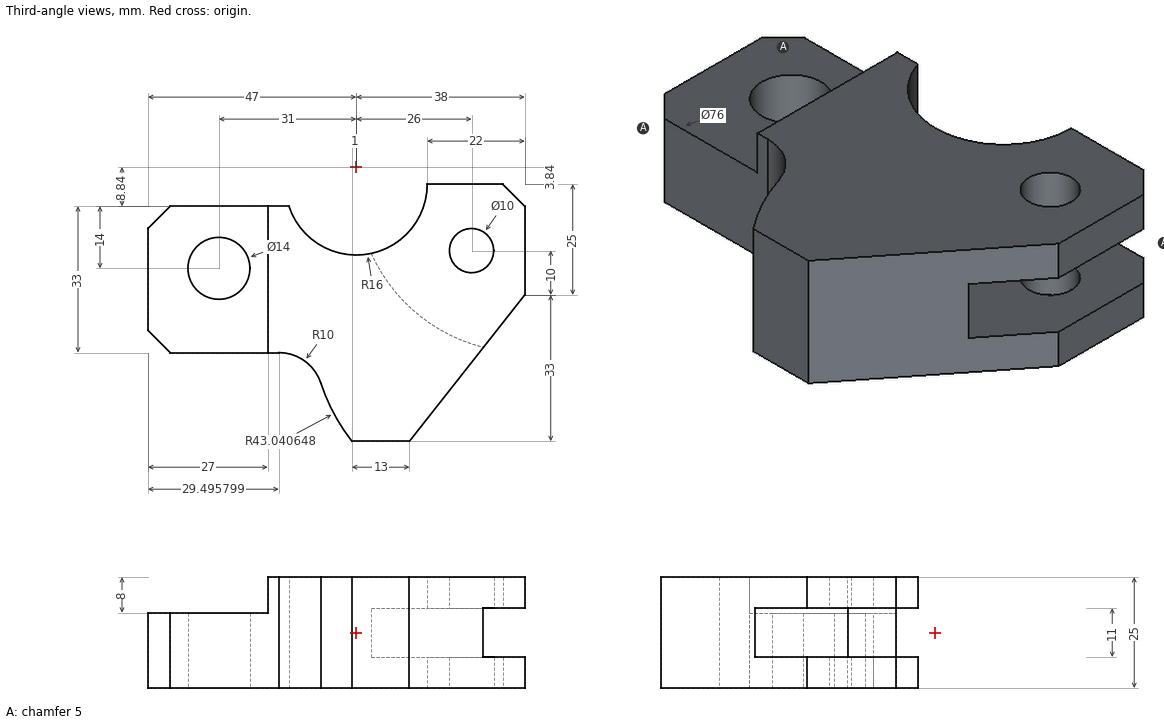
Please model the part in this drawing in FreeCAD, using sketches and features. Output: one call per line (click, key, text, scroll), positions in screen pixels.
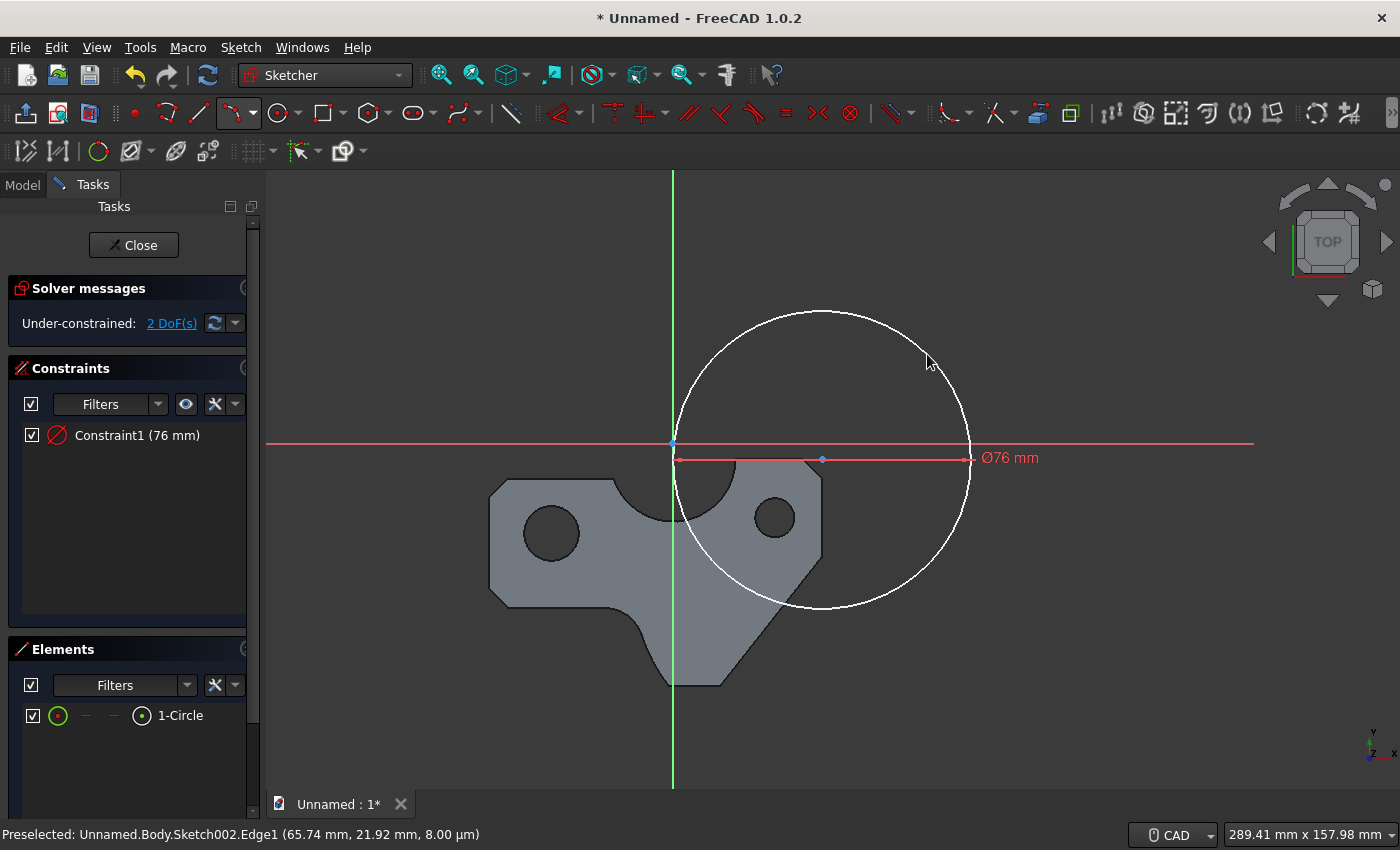
key(d)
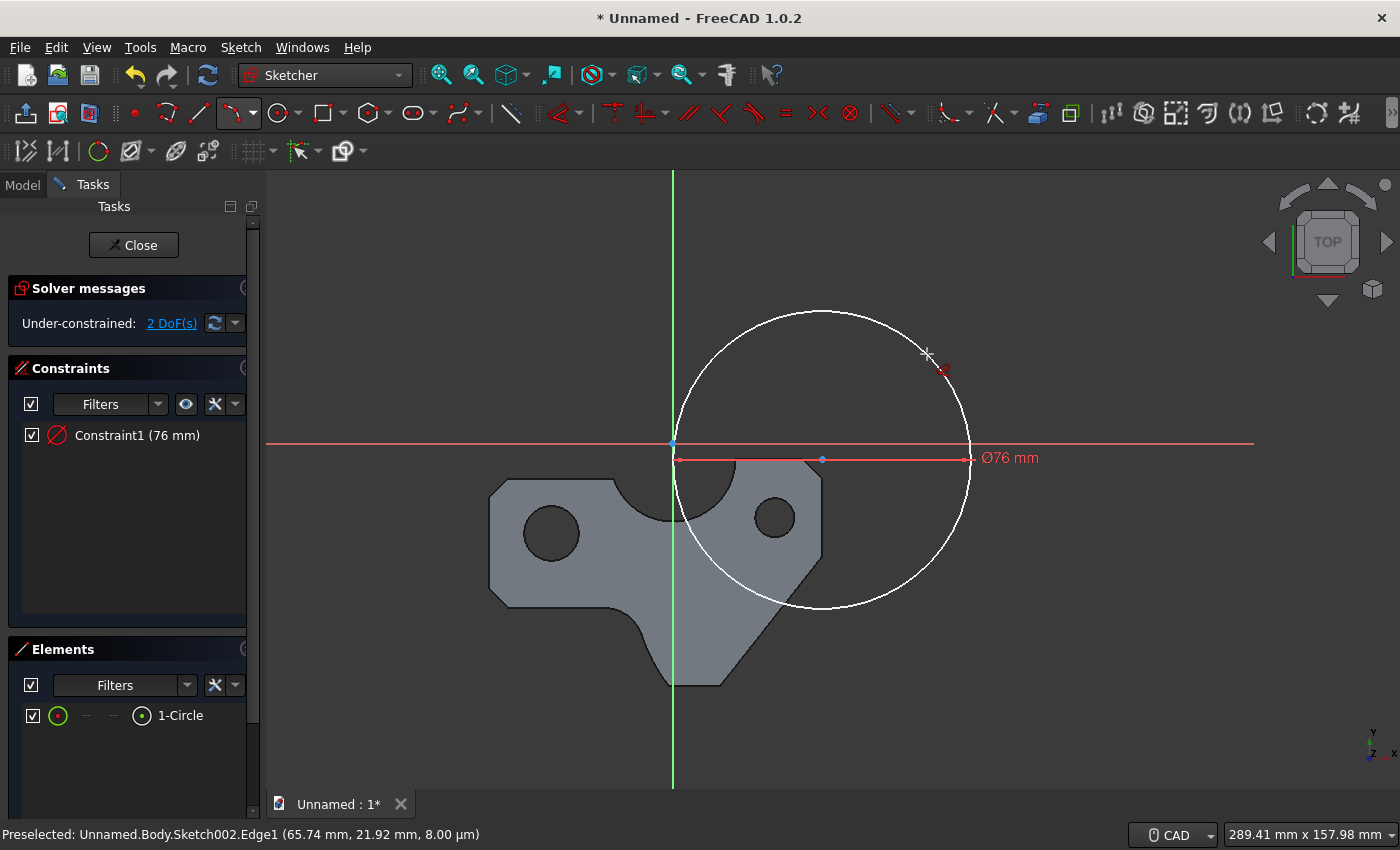
click(822, 460)
click(747, 410)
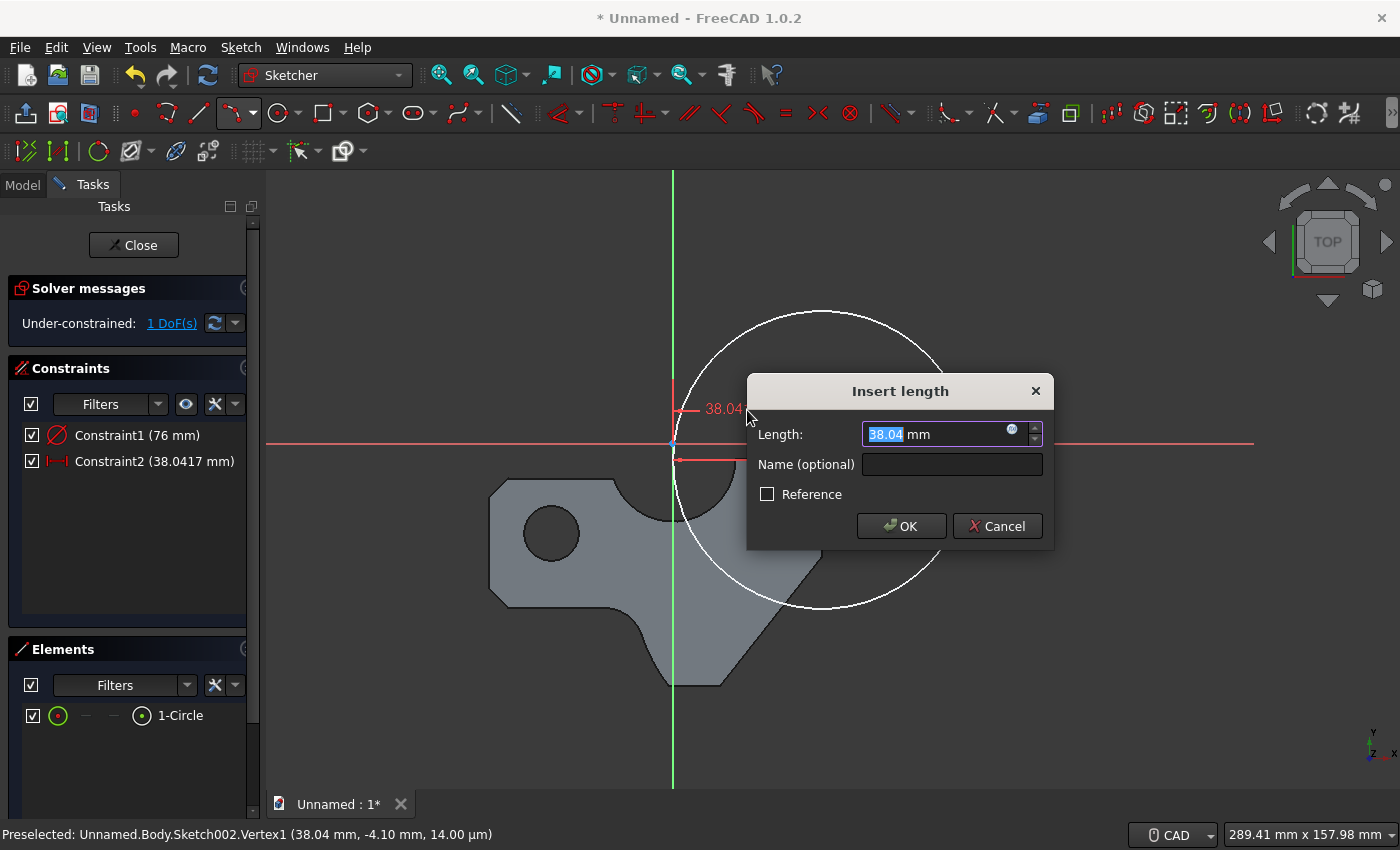
text(38)
key(Return)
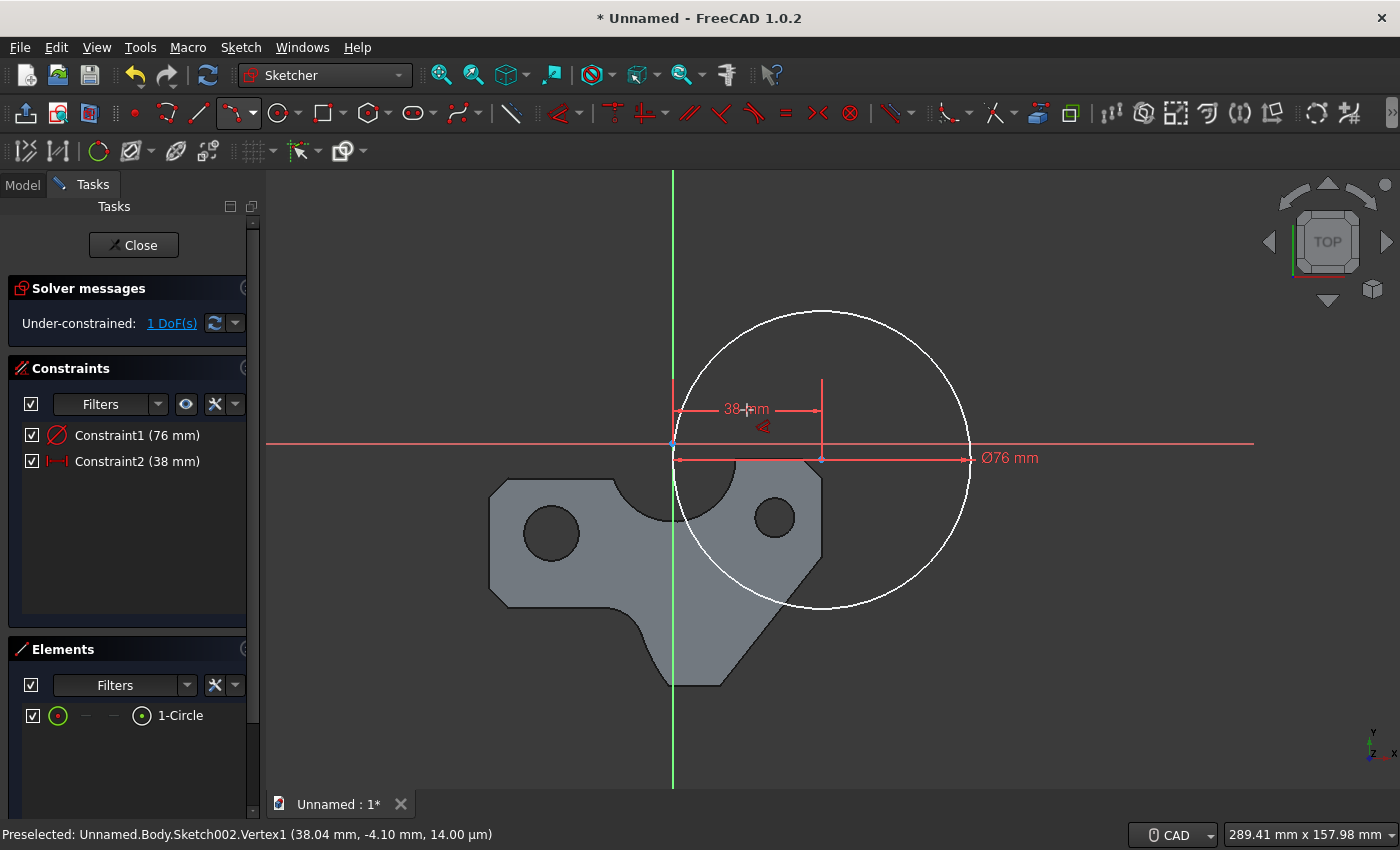
scroll(822, 460, up, 5)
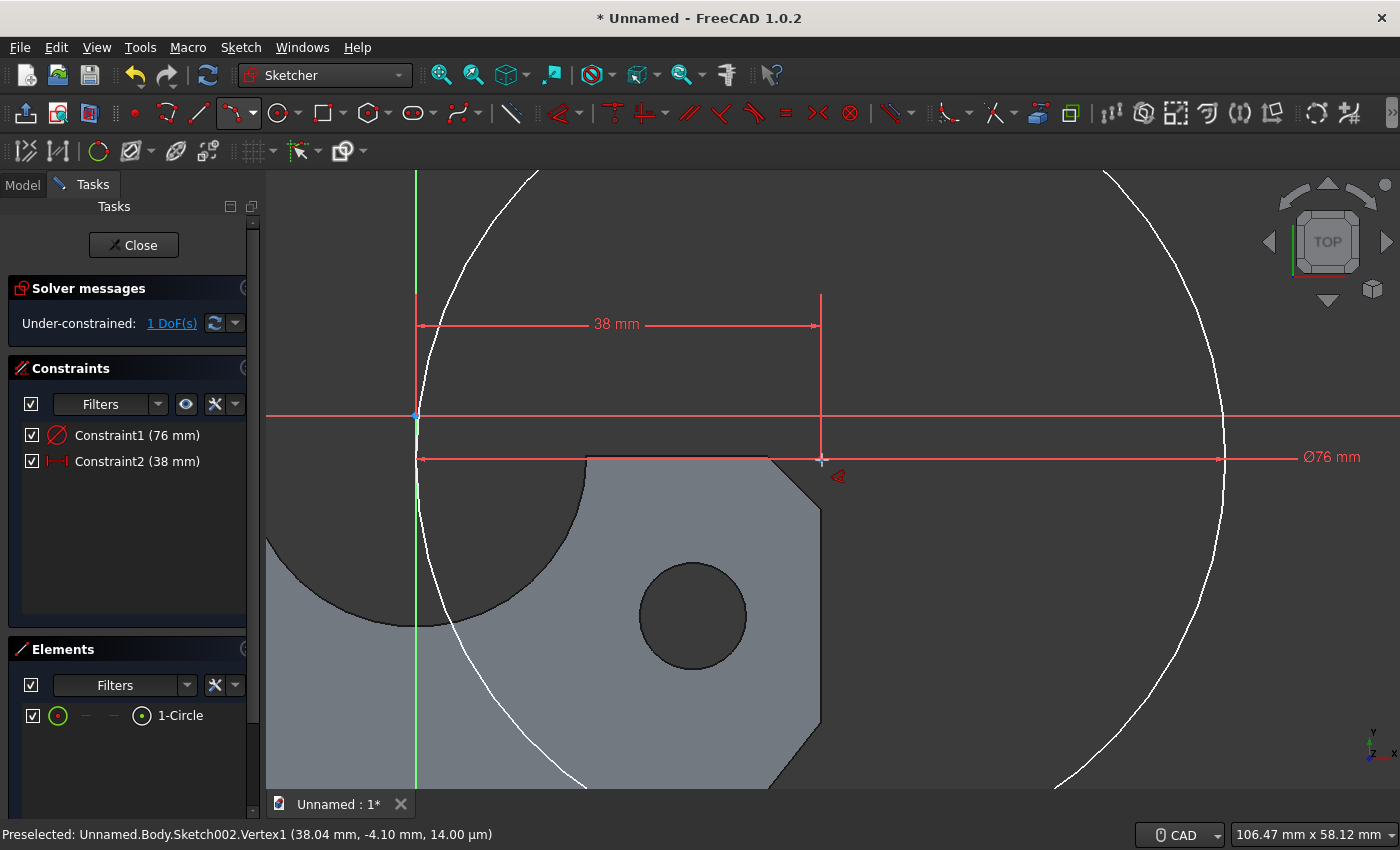
click(821, 459)
click(382, 437)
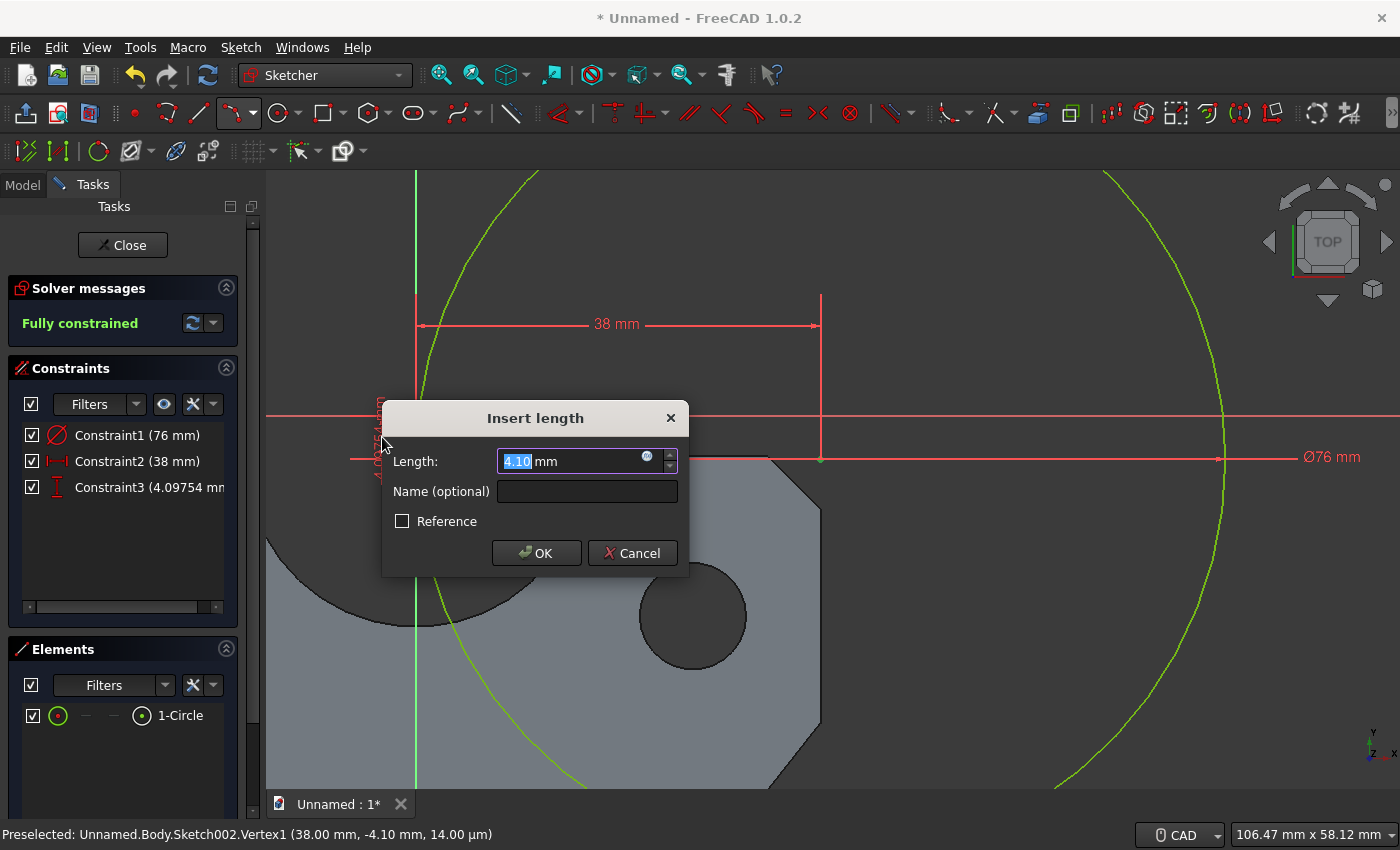
text(3.84)
key(Return)
key(Escape)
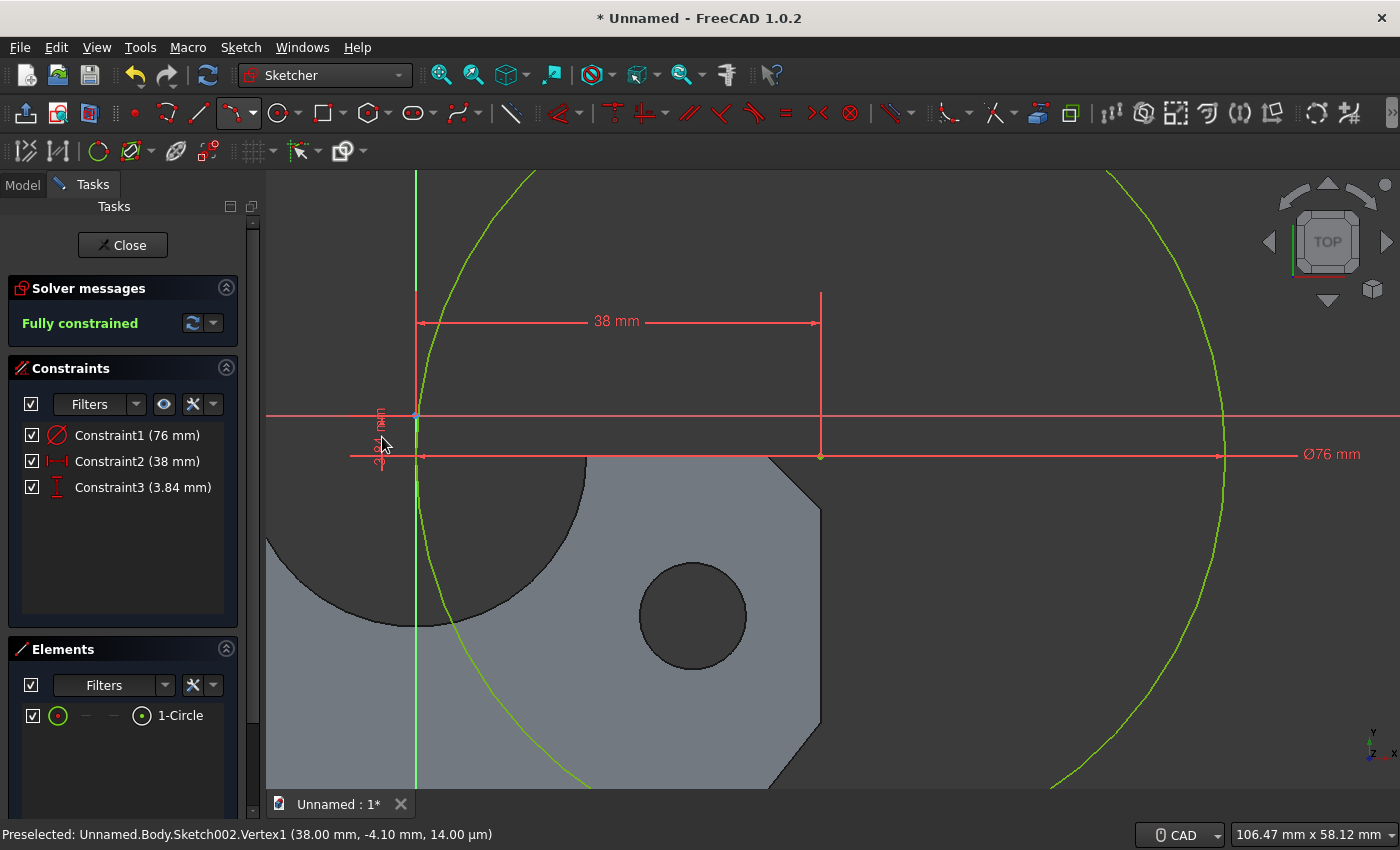
click(123, 245)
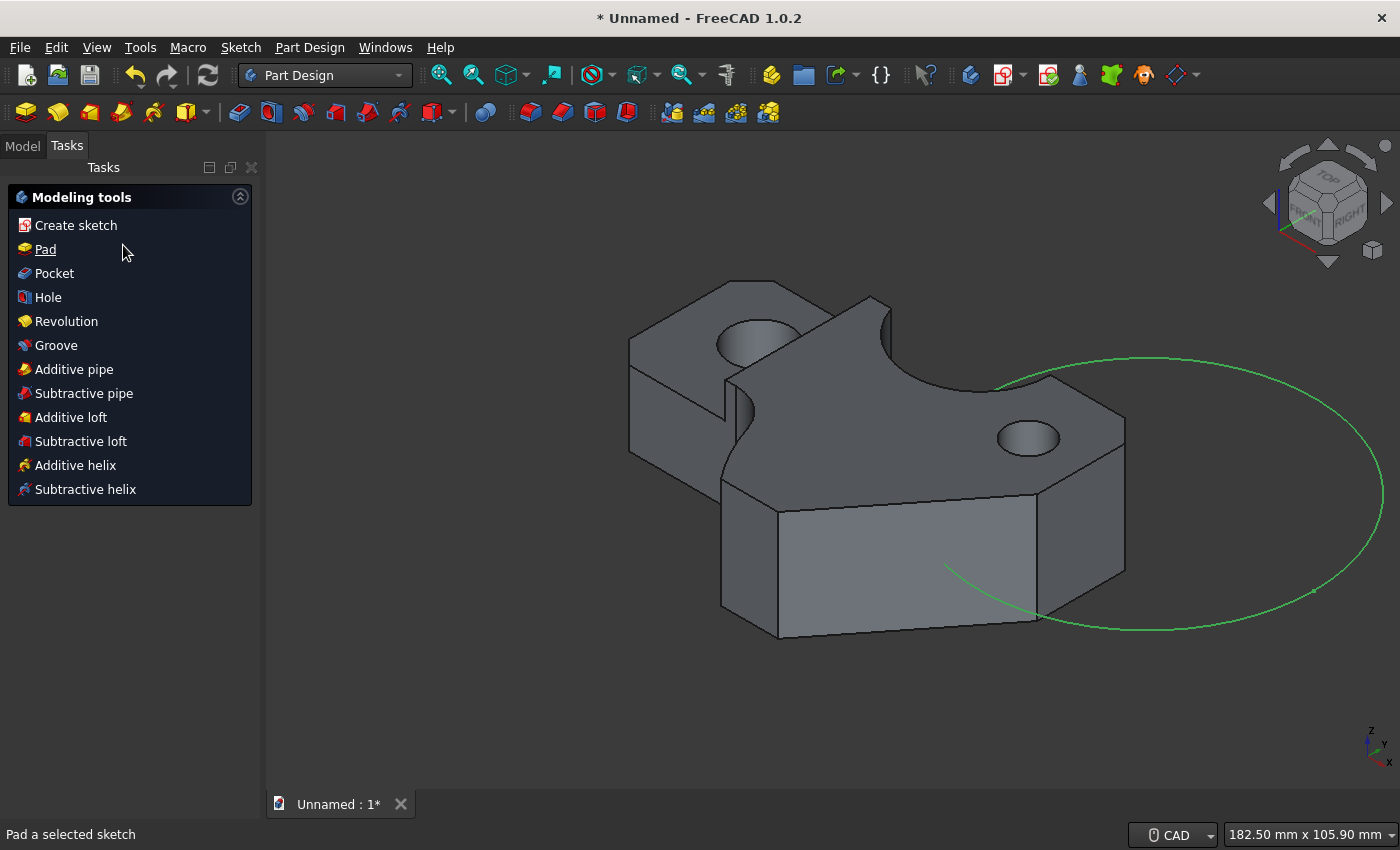
click(240, 112)